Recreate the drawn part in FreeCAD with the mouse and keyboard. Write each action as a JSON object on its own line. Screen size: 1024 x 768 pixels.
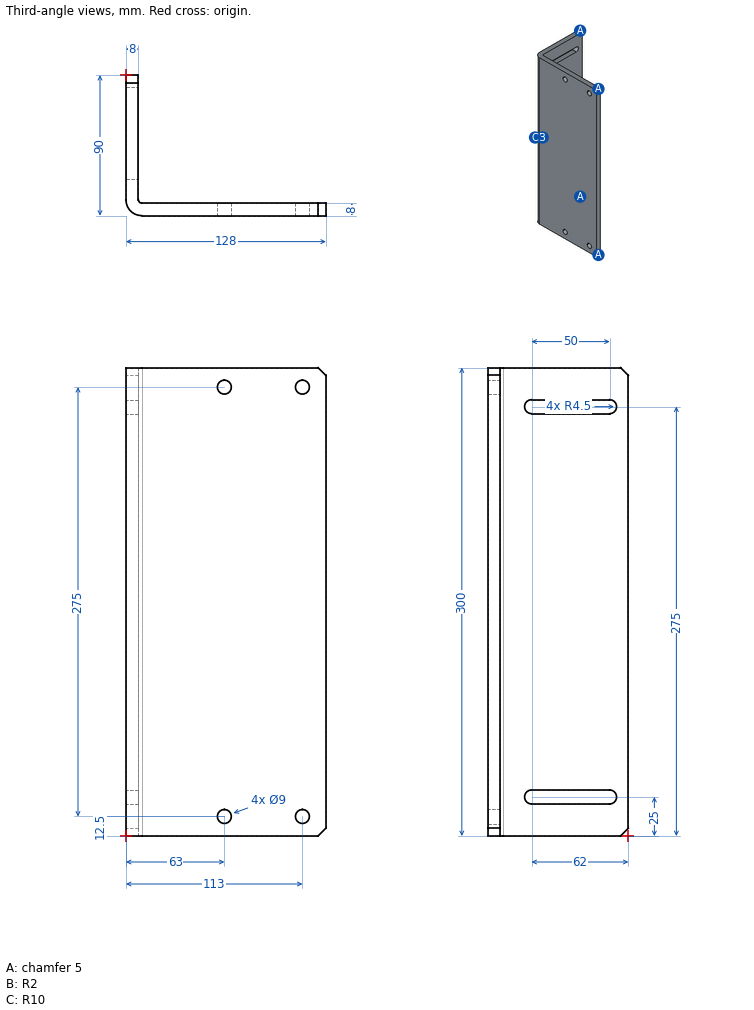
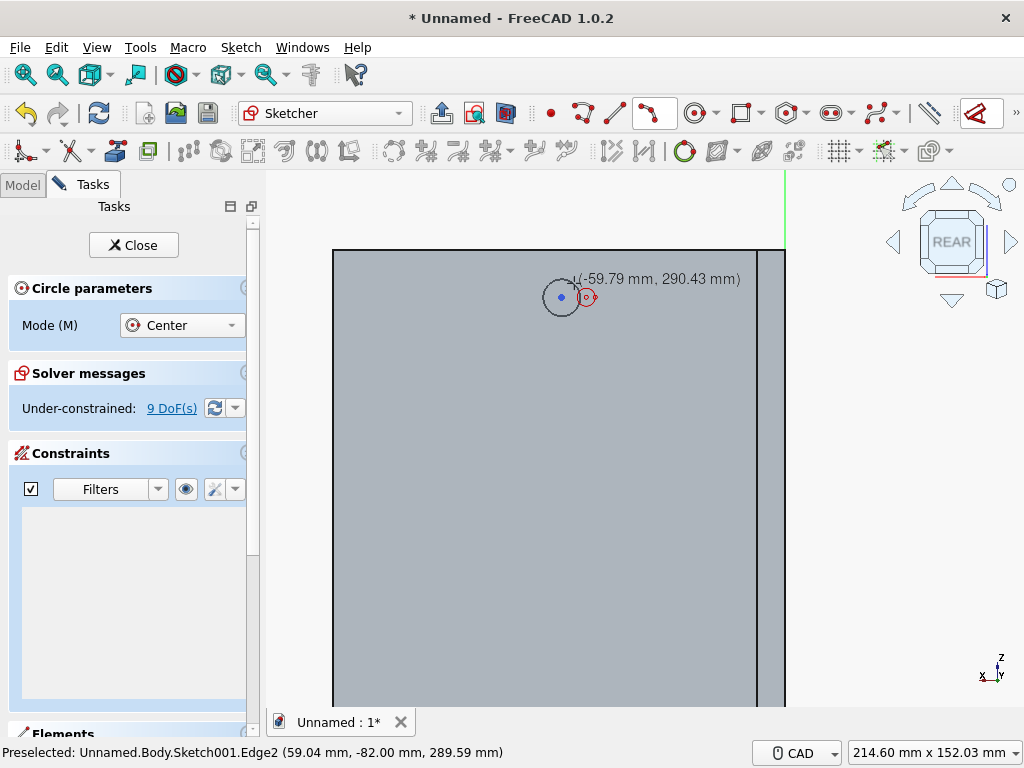
{"action": "scroll", "coordinate": [386, 294], "scroll_direction": "up", "scroll_amount": 2}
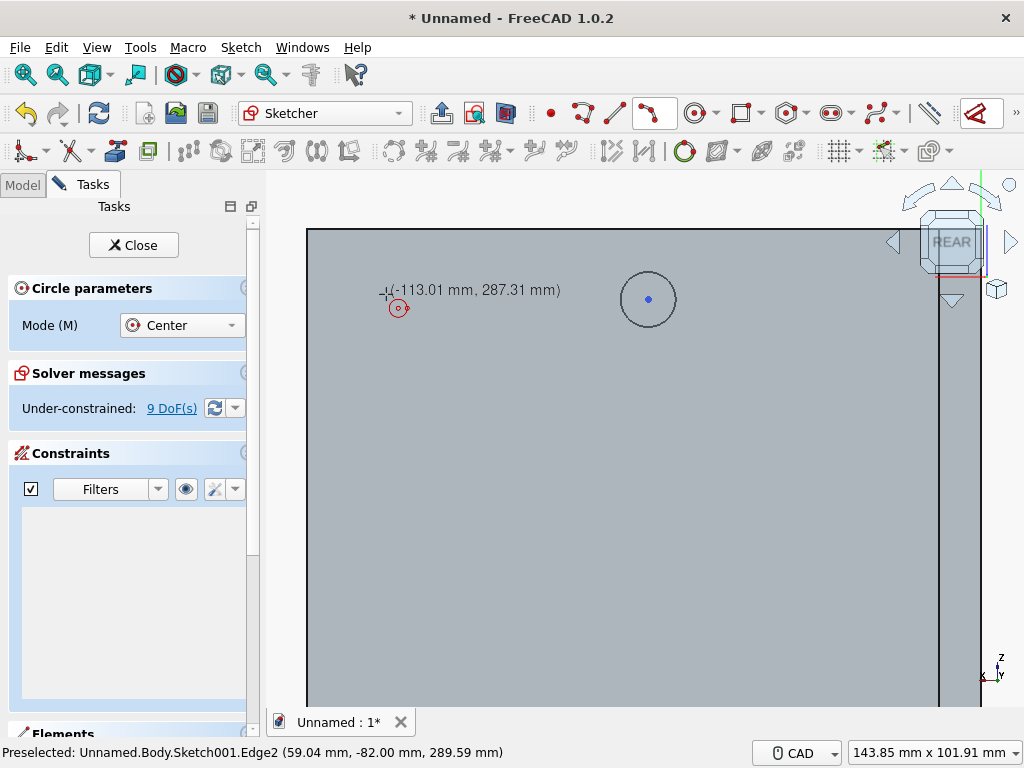
{"action": "scroll", "coordinate": [552, 286], "scroll_direction": "down", "scroll_amount": 8}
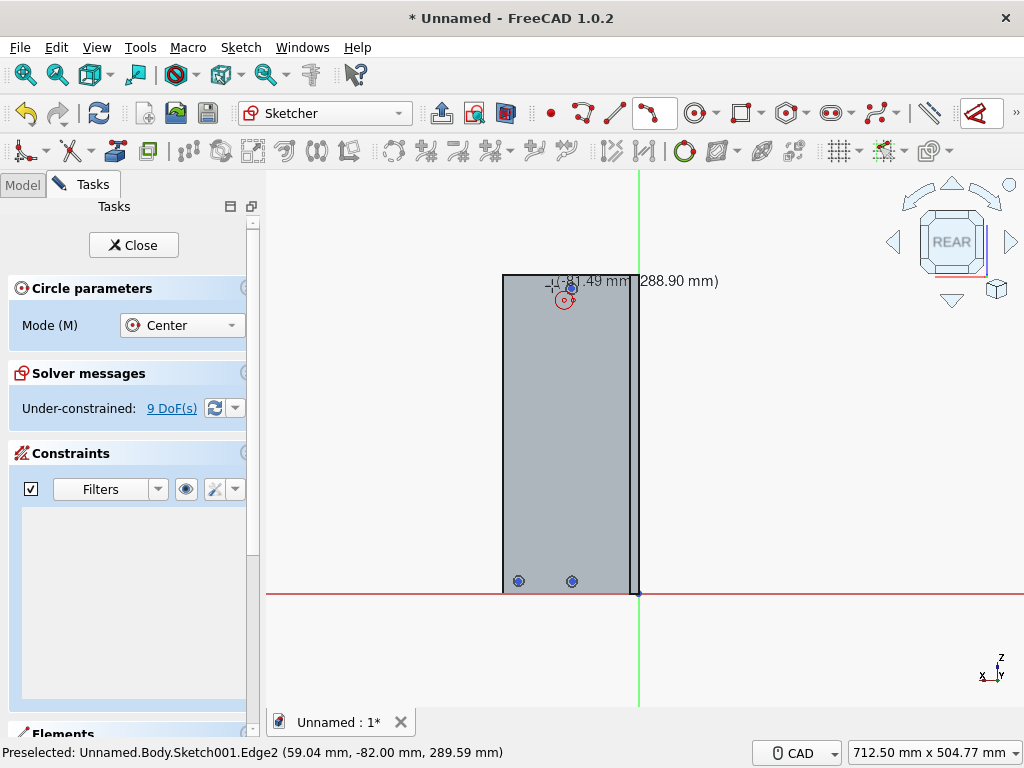
{"action": "left_click", "coordinate": [519, 288]}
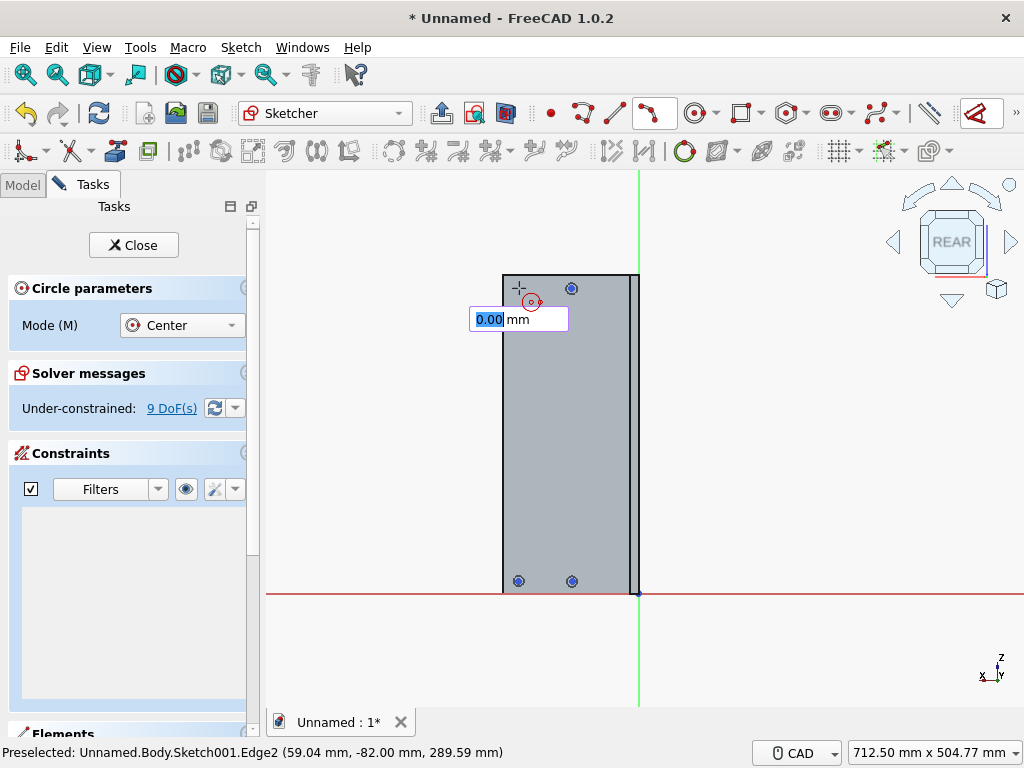
{"action": "scroll", "coordinate": [522, 284], "scroll_direction": "up", "scroll_amount": 6}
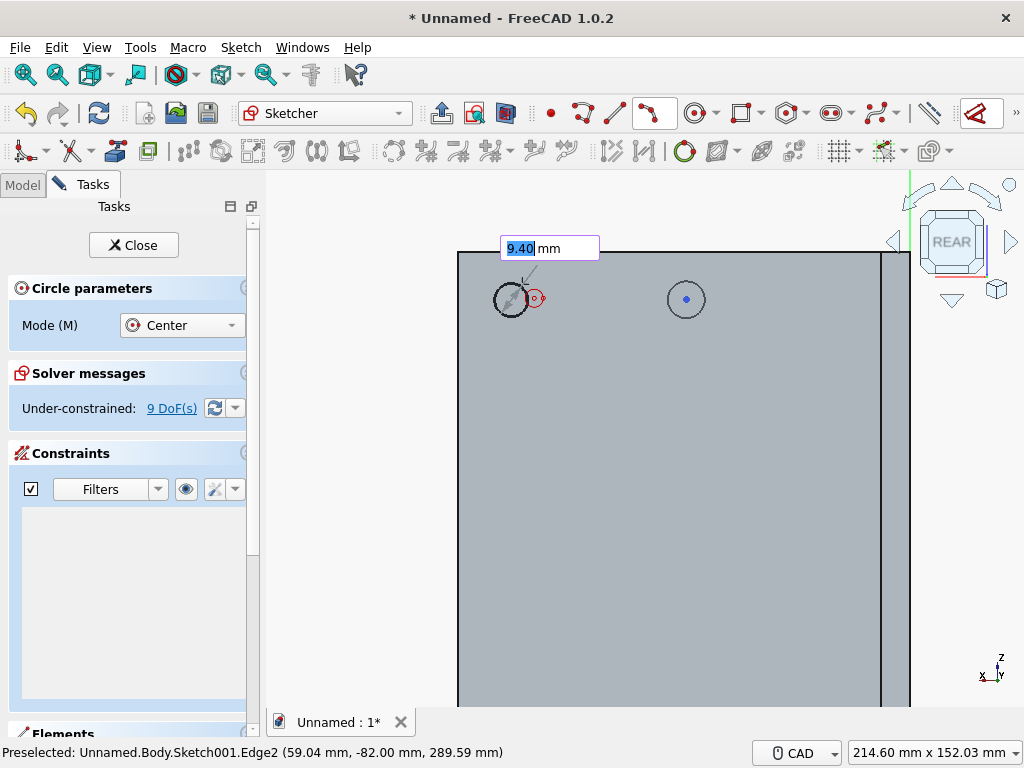
{"action": "left_click", "coordinate": [522, 285]}
{"action": "key", "text": "Escape"}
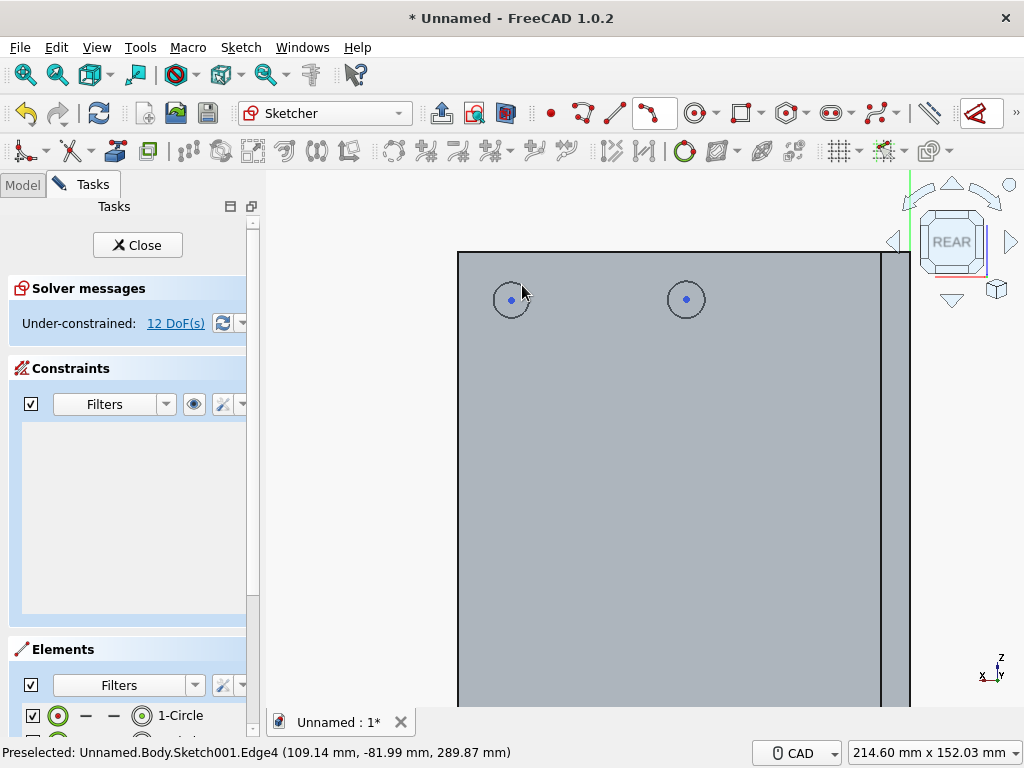
{"action": "scroll", "coordinate": [522, 284], "scroll_direction": "down", "scroll_amount": 6}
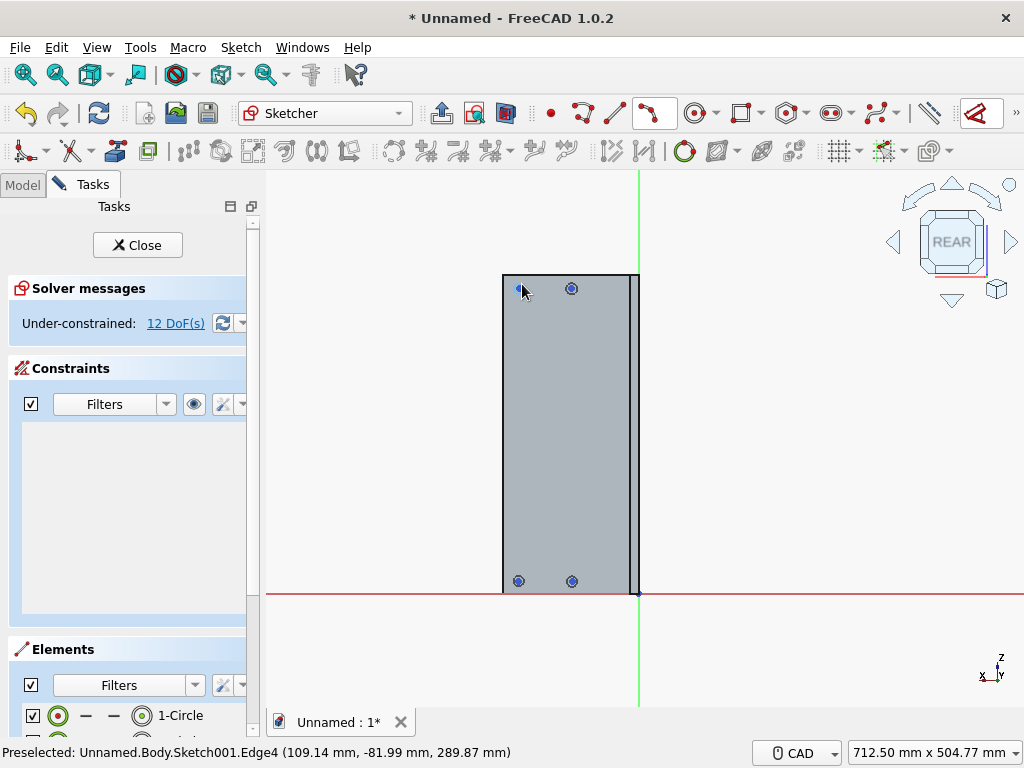
{"action": "scroll", "coordinate": [576, 578], "scroll_direction": "up", "scroll_amount": 5}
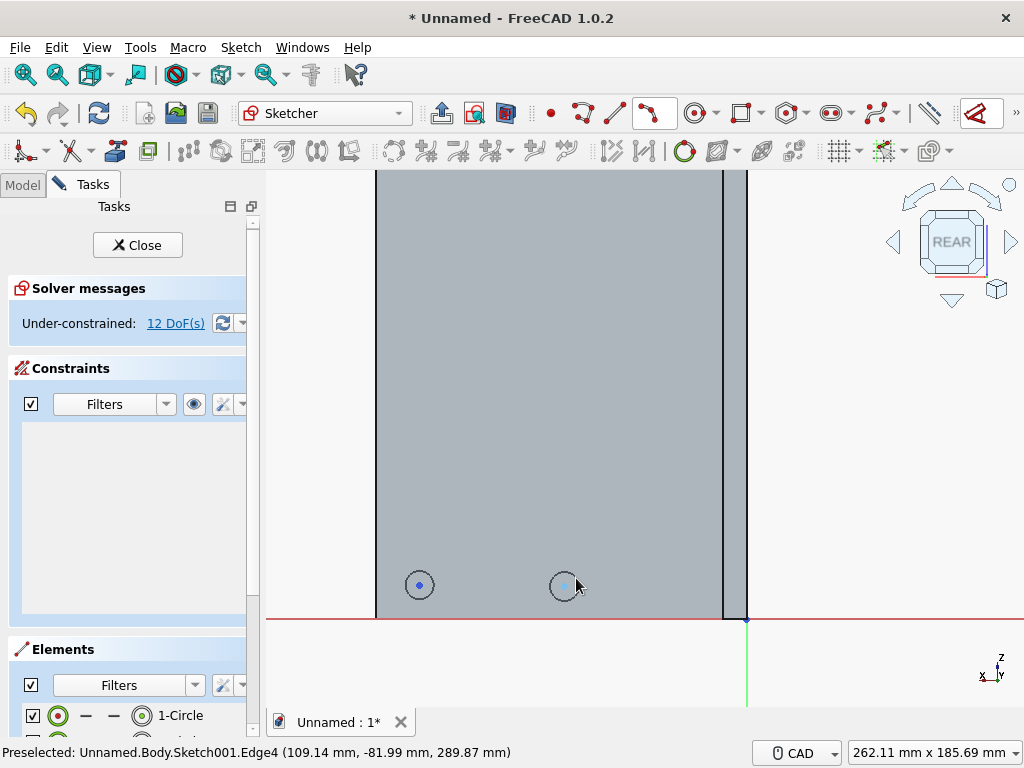
{"action": "left_click", "coordinate": [575, 576]}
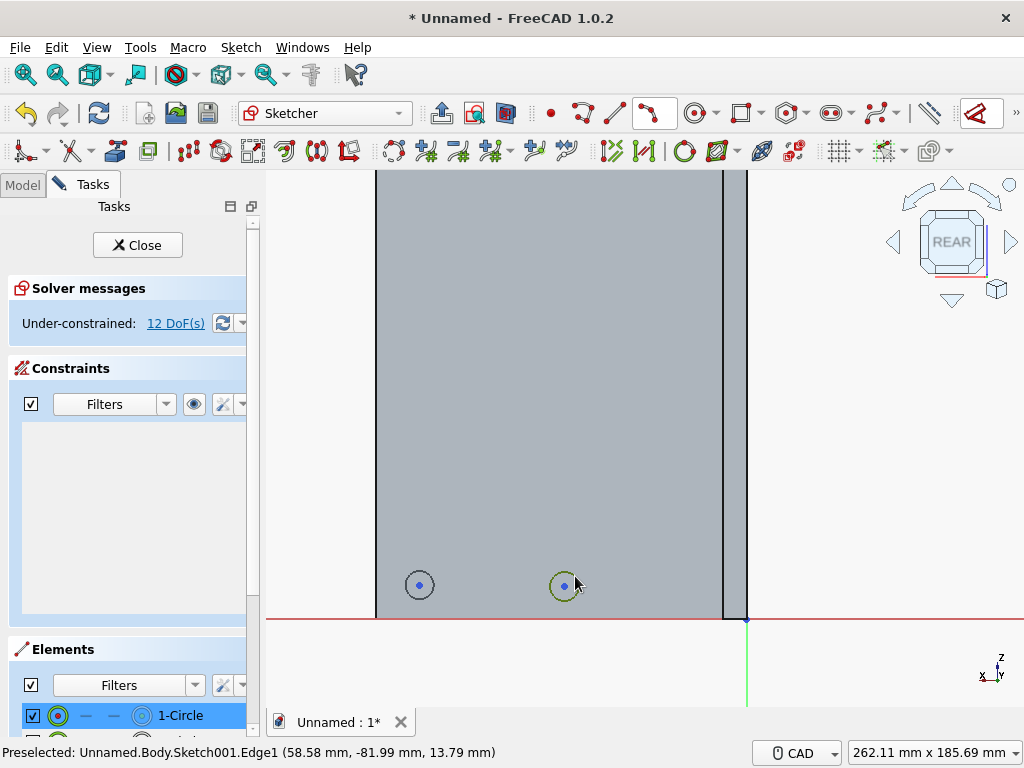
{"action": "left_click", "coordinate": [429, 575]}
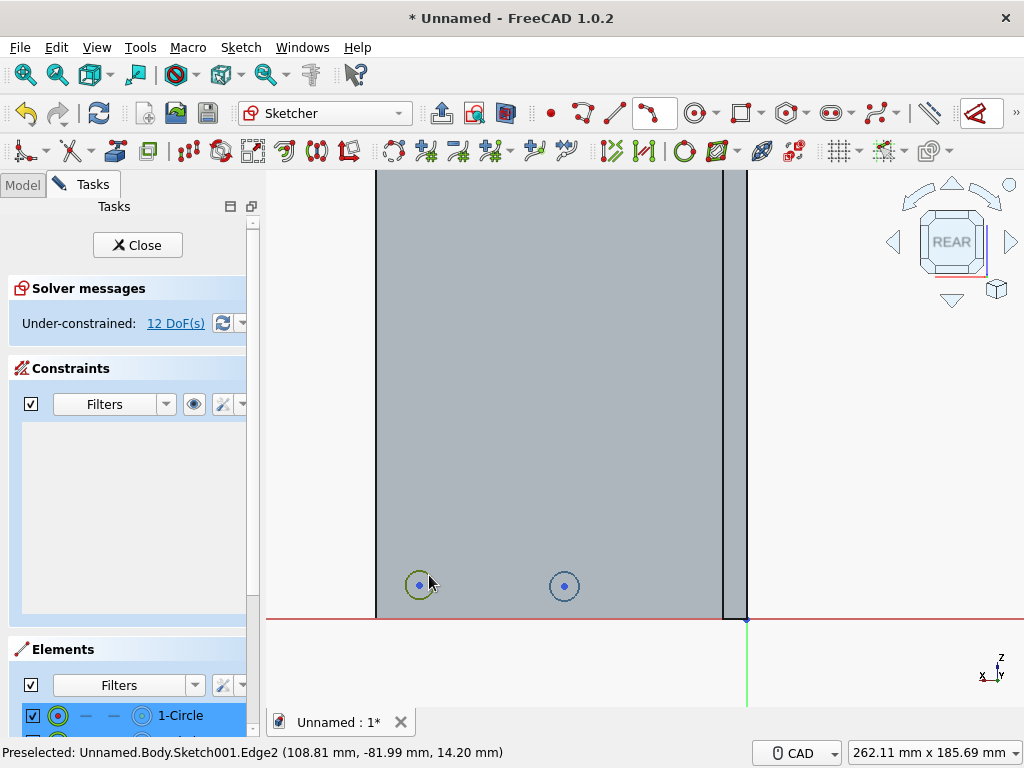
{"action": "scroll", "coordinate": [576, 579], "scroll_direction": "down", "scroll_amount": 5}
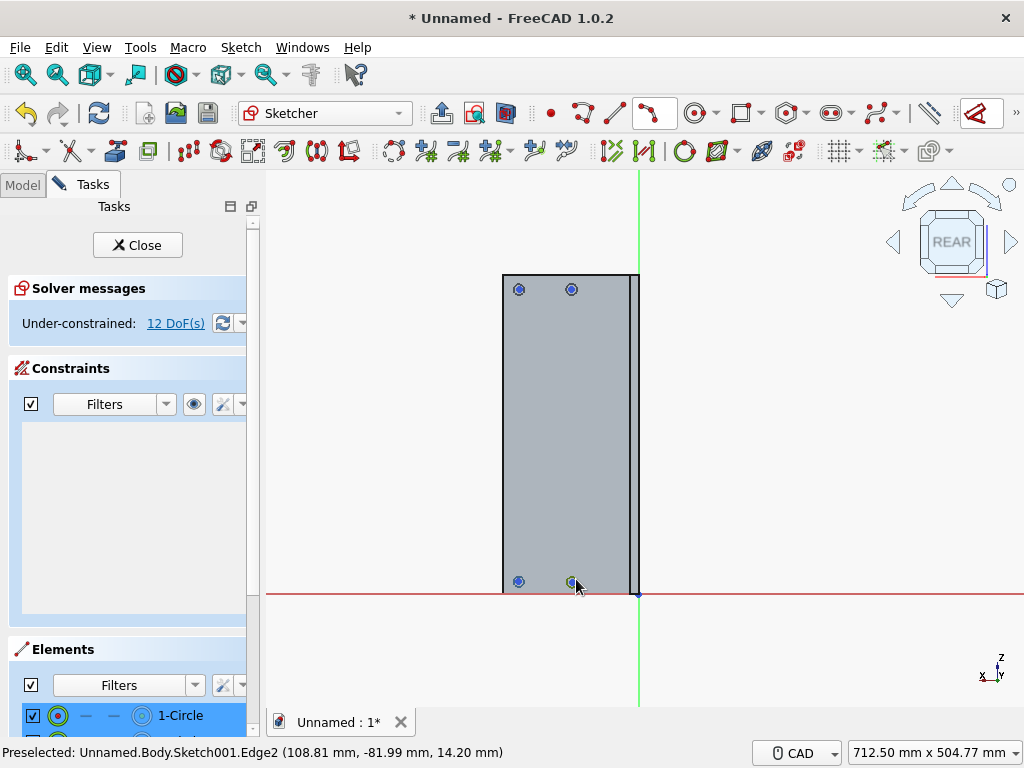
{"action": "scroll", "coordinate": [576, 286], "scroll_direction": "up", "scroll_amount": 5}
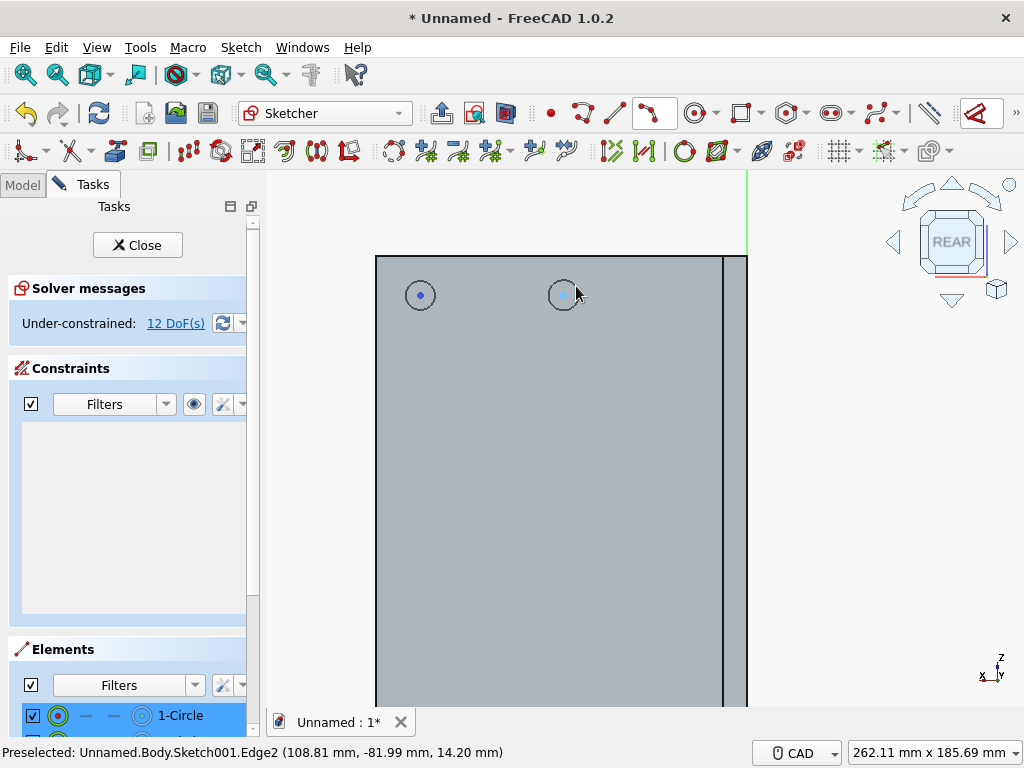
{"action": "left_click", "coordinate": [574, 285]}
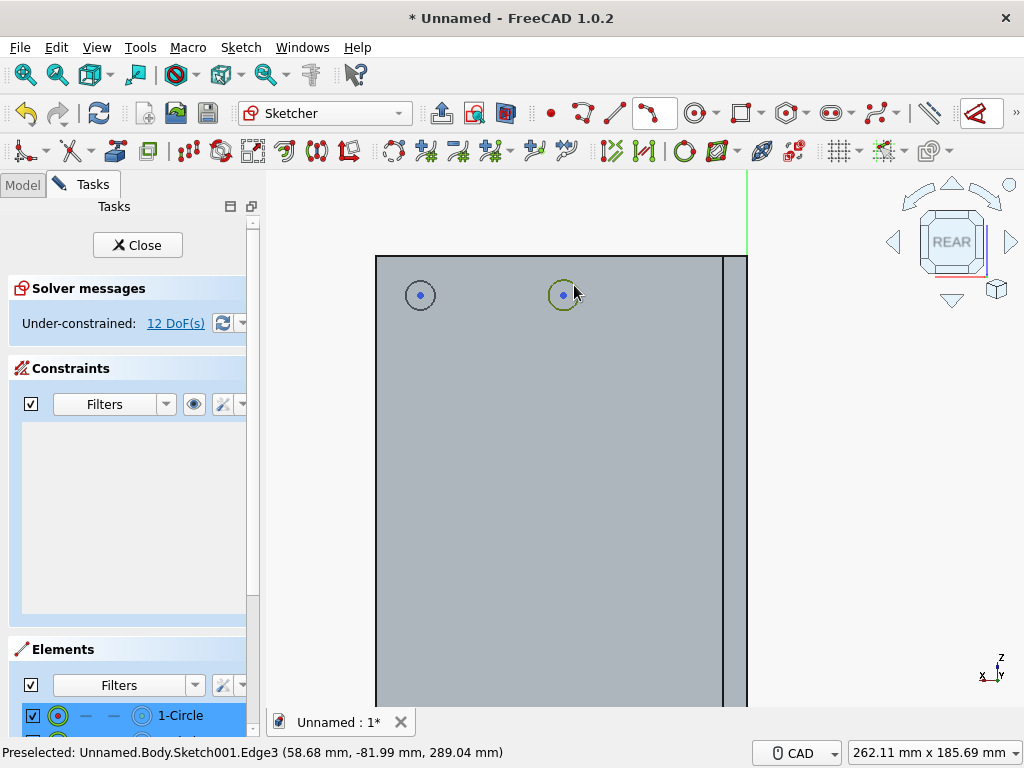
{"action": "left_click", "coordinate": [431, 285]}